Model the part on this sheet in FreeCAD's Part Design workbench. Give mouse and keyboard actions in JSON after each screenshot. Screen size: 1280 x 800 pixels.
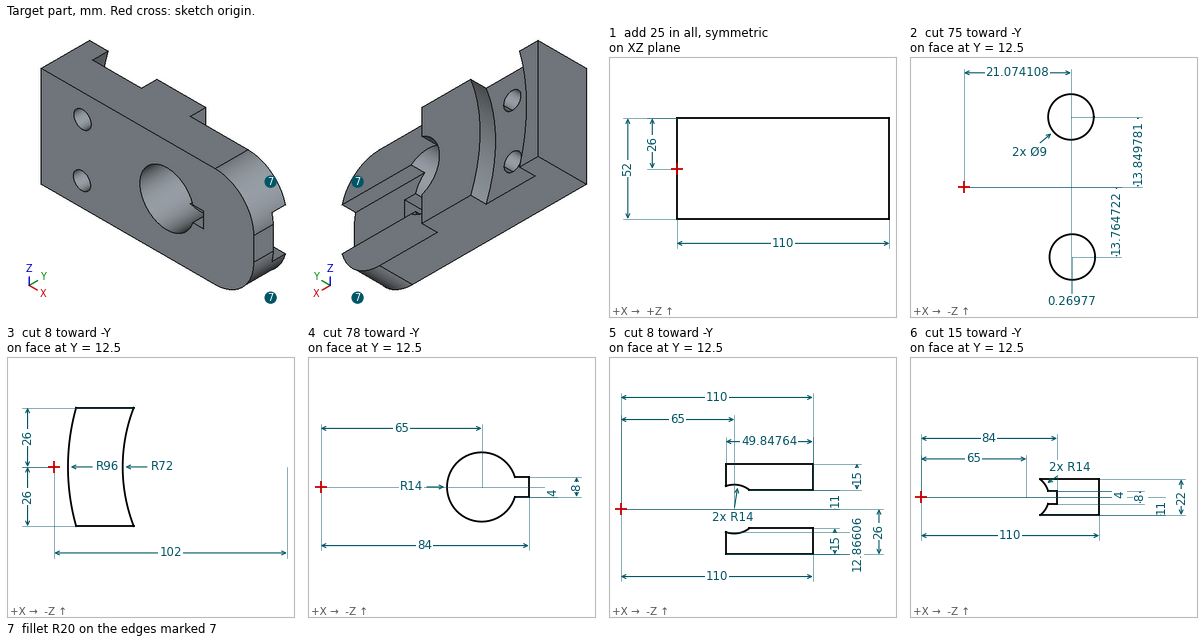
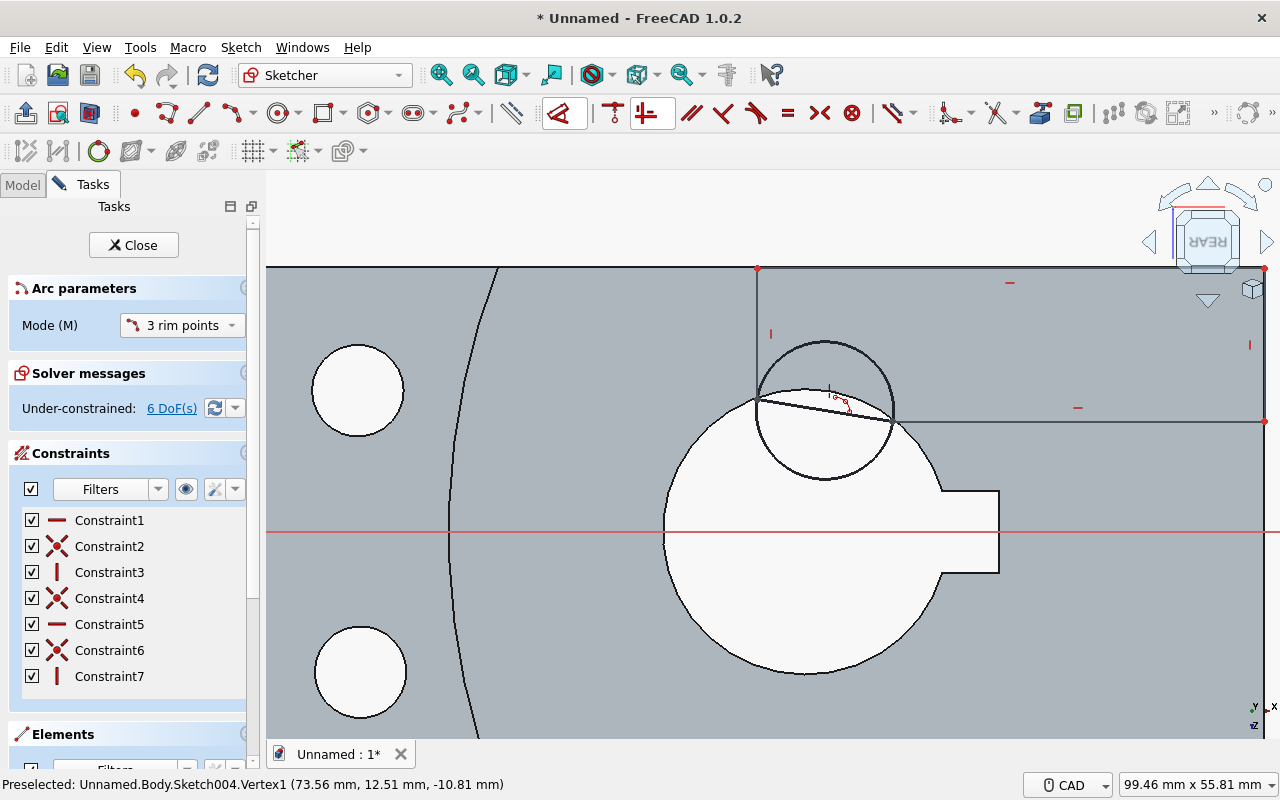
{"action": "left_click", "coordinate": [828, 391]}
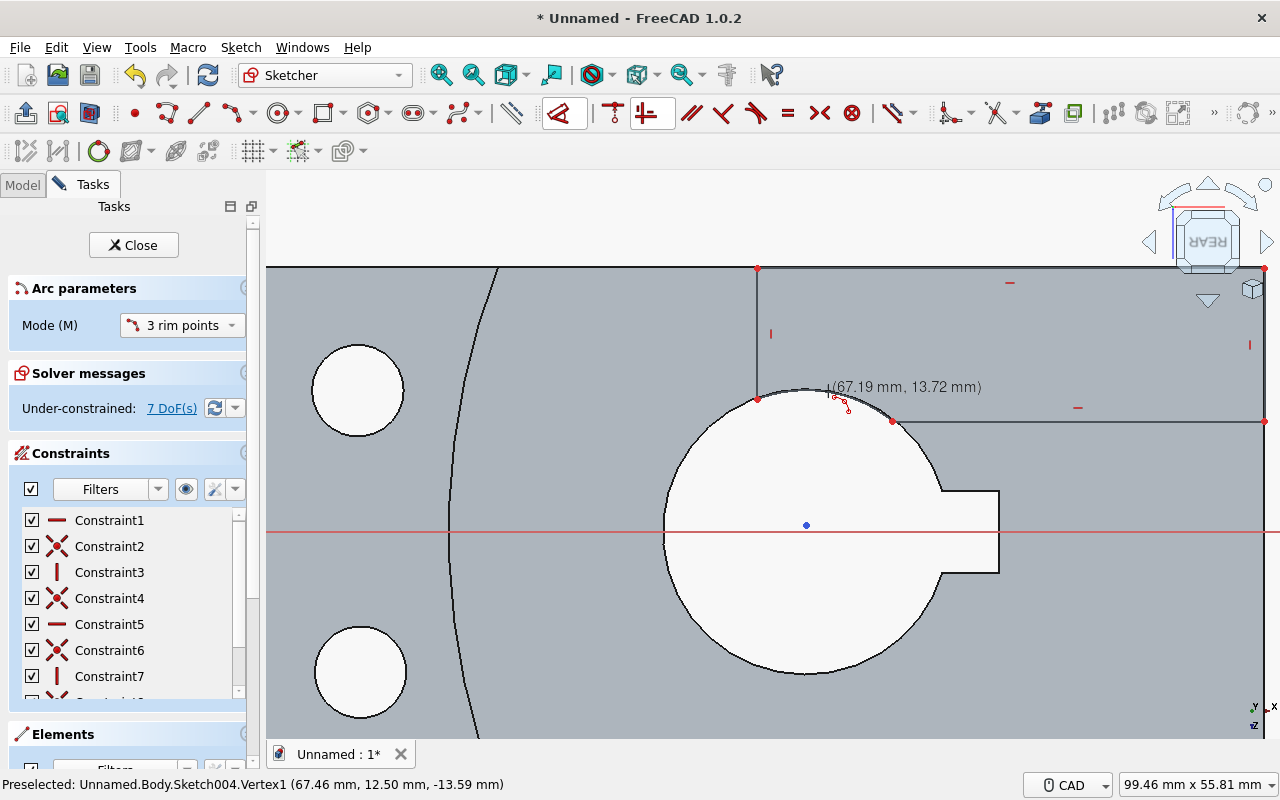
{"action": "left_click", "coordinate": [168, 114]}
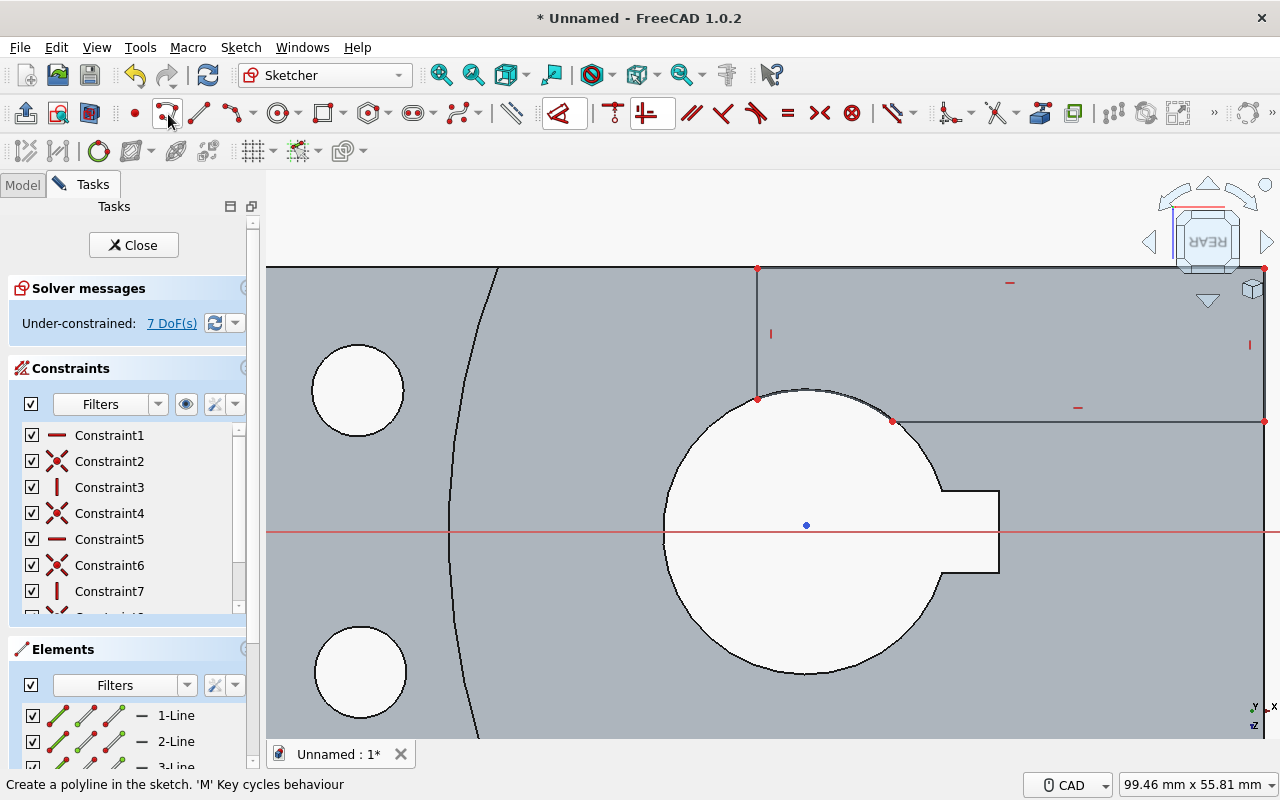
{"action": "left_click", "coordinate": [756, 666]}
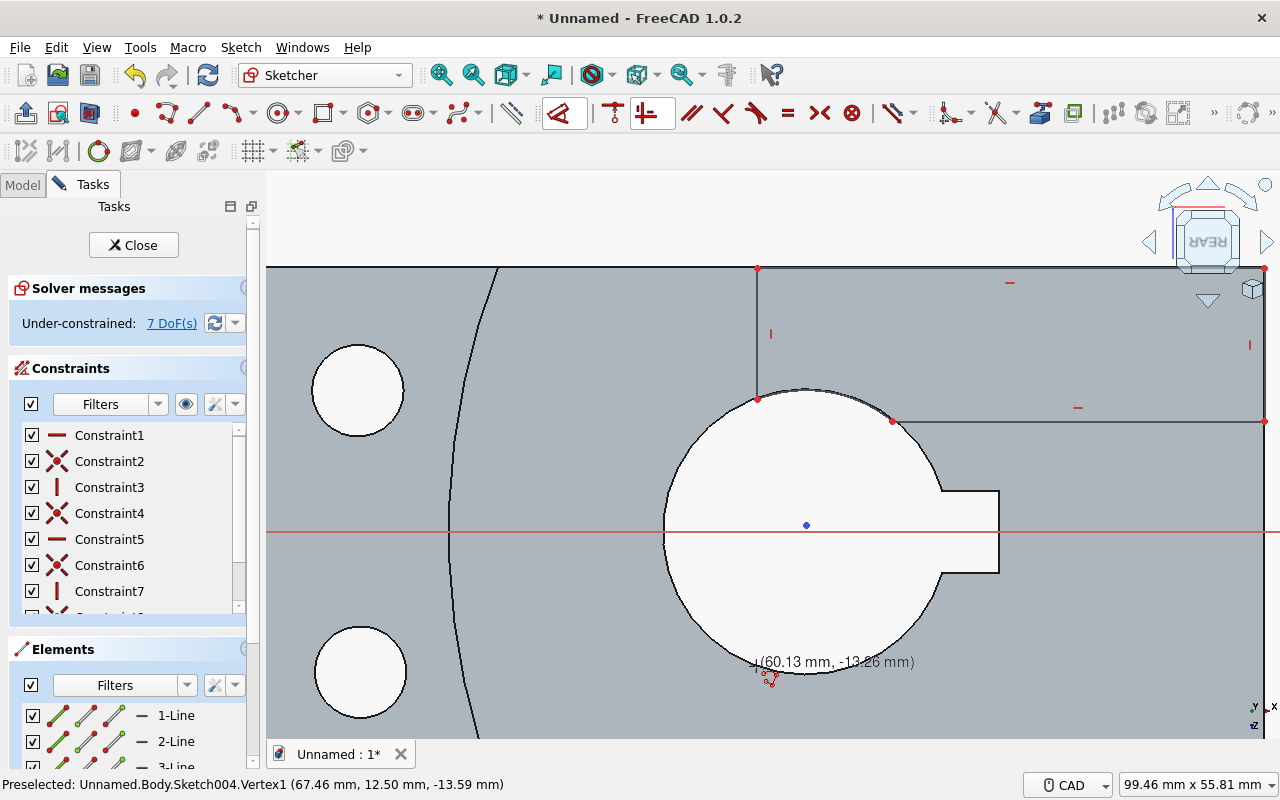
{"action": "scroll", "coordinate": [705, 360], "scroll_direction": "down", "scroll_amount": 3}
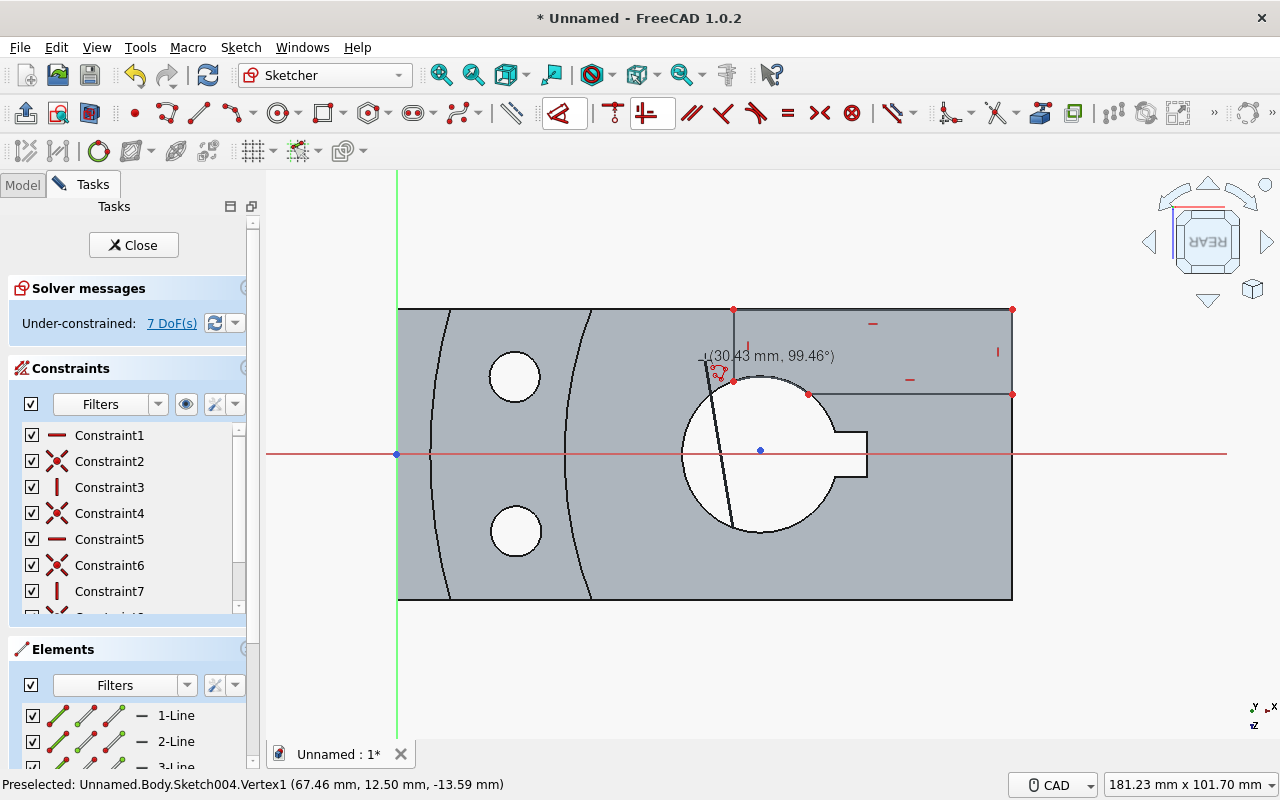
{"action": "left_click", "coordinate": [733, 600]}
{"action": "left_click", "coordinate": [1012, 600]}
{"action": "left_click", "coordinate": [1012, 516]}
{"action": "left_click", "coordinate": [809, 516]}
{"action": "right_click", "coordinate": [809, 516]}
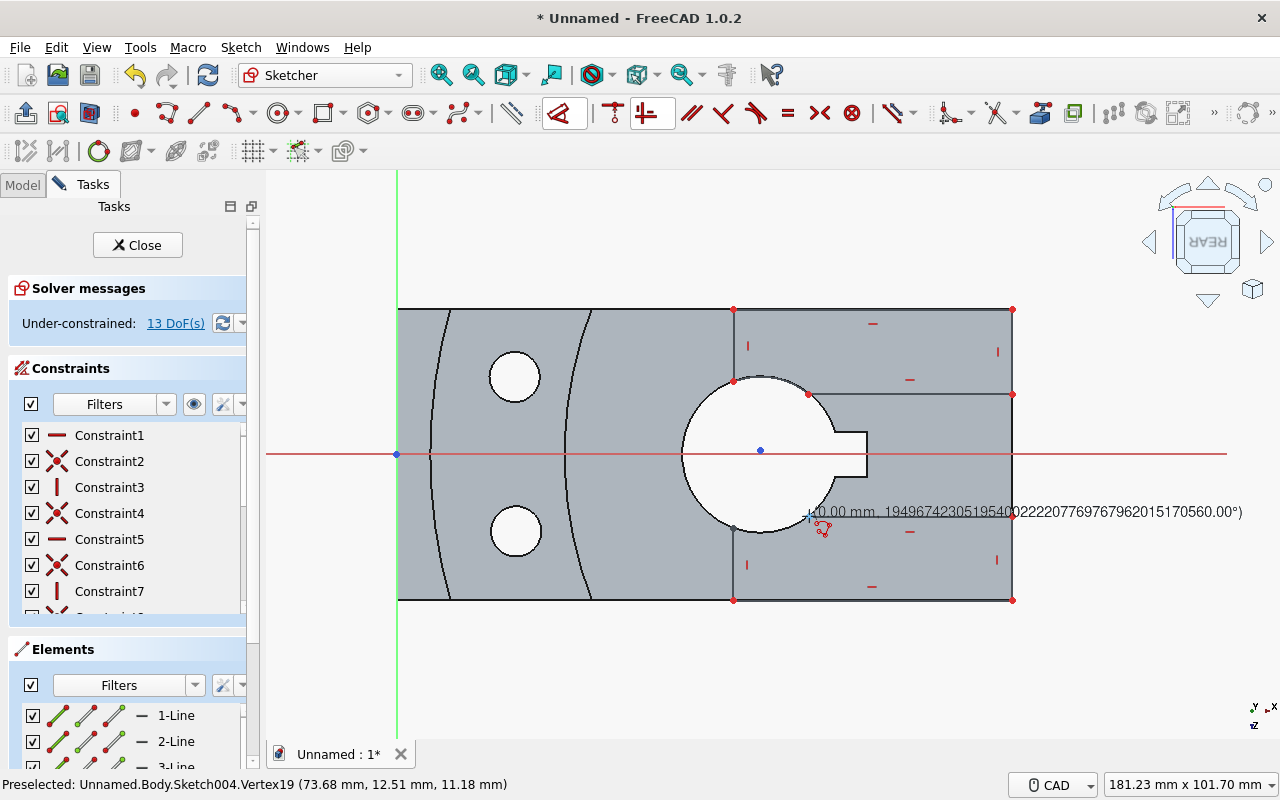
{"action": "left_click", "coordinate": [232, 114]}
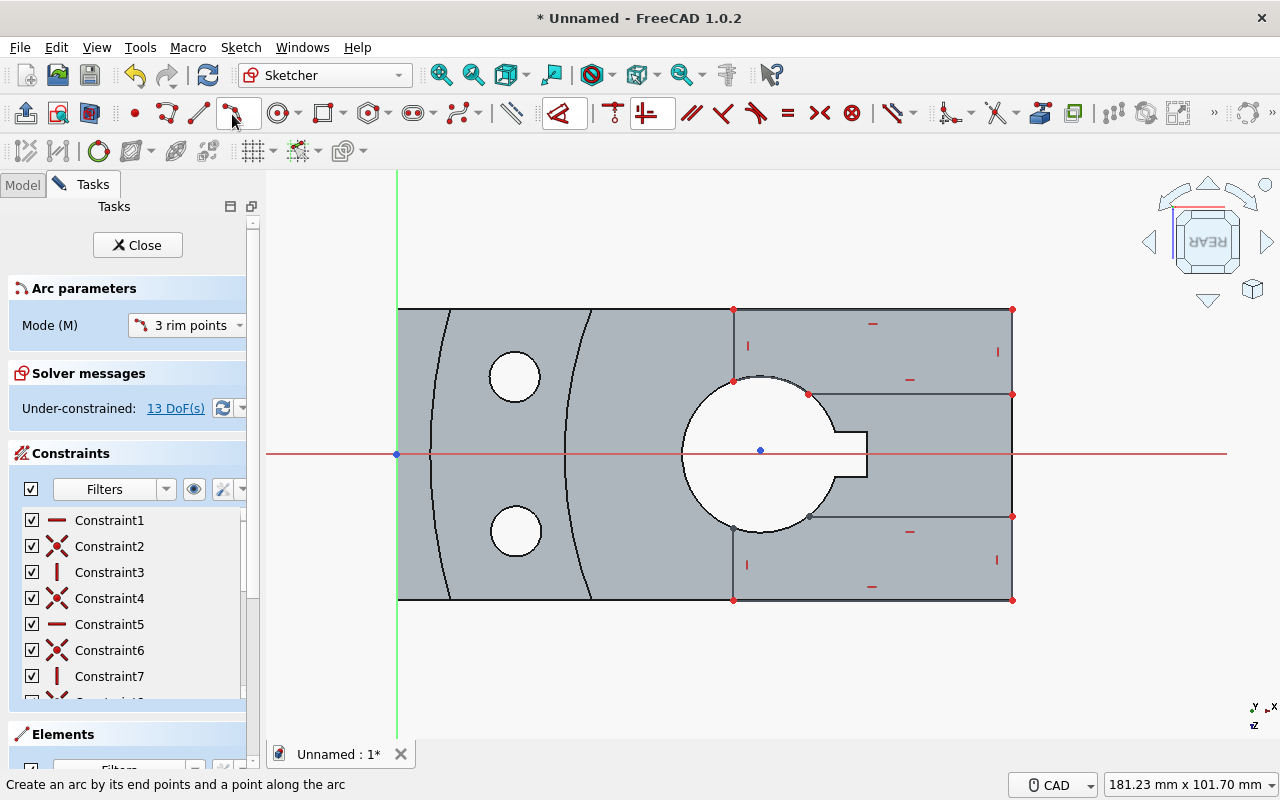
{"action": "left_click", "coordinate": [809, 517]}
{"action": "left_click", "coordinate": [733, 529]}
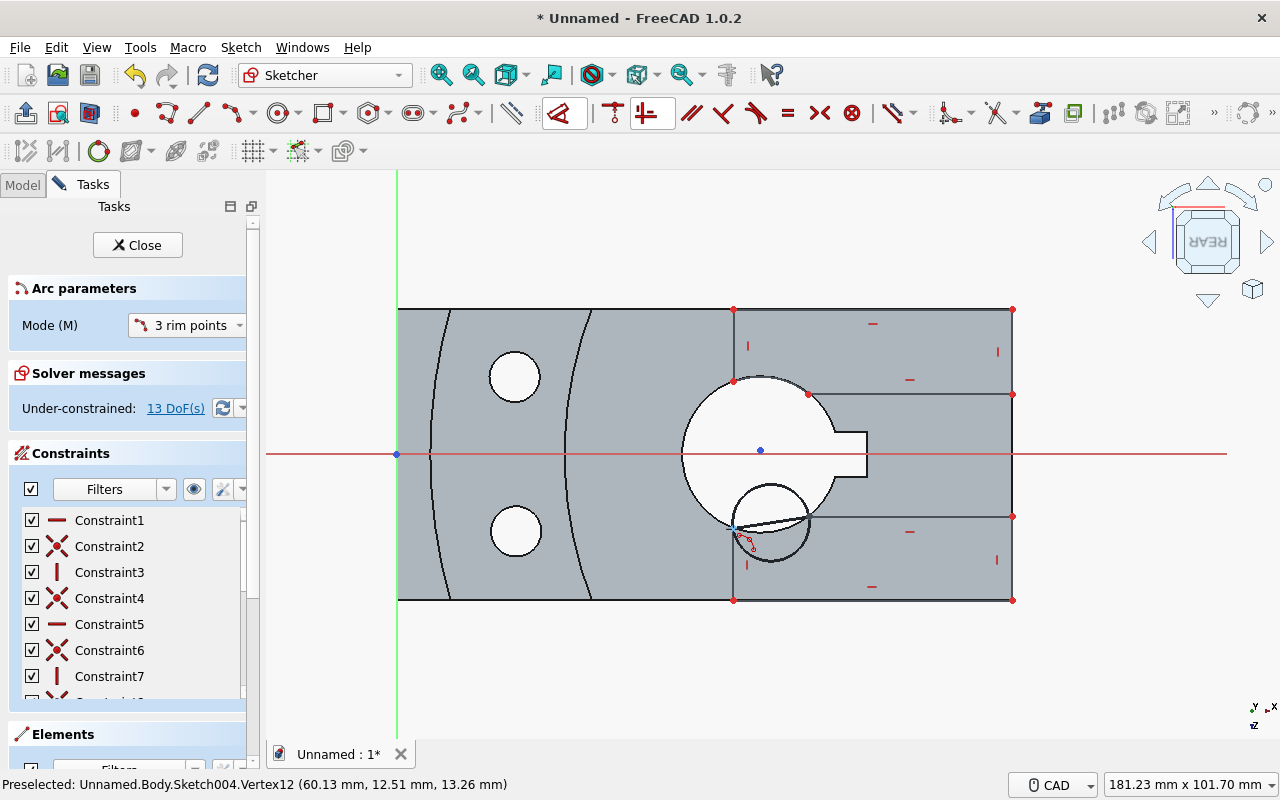
{"action": "scroll", "coordinate": [773, 532], "scroll_direction": "up", "scroll_amount": 3}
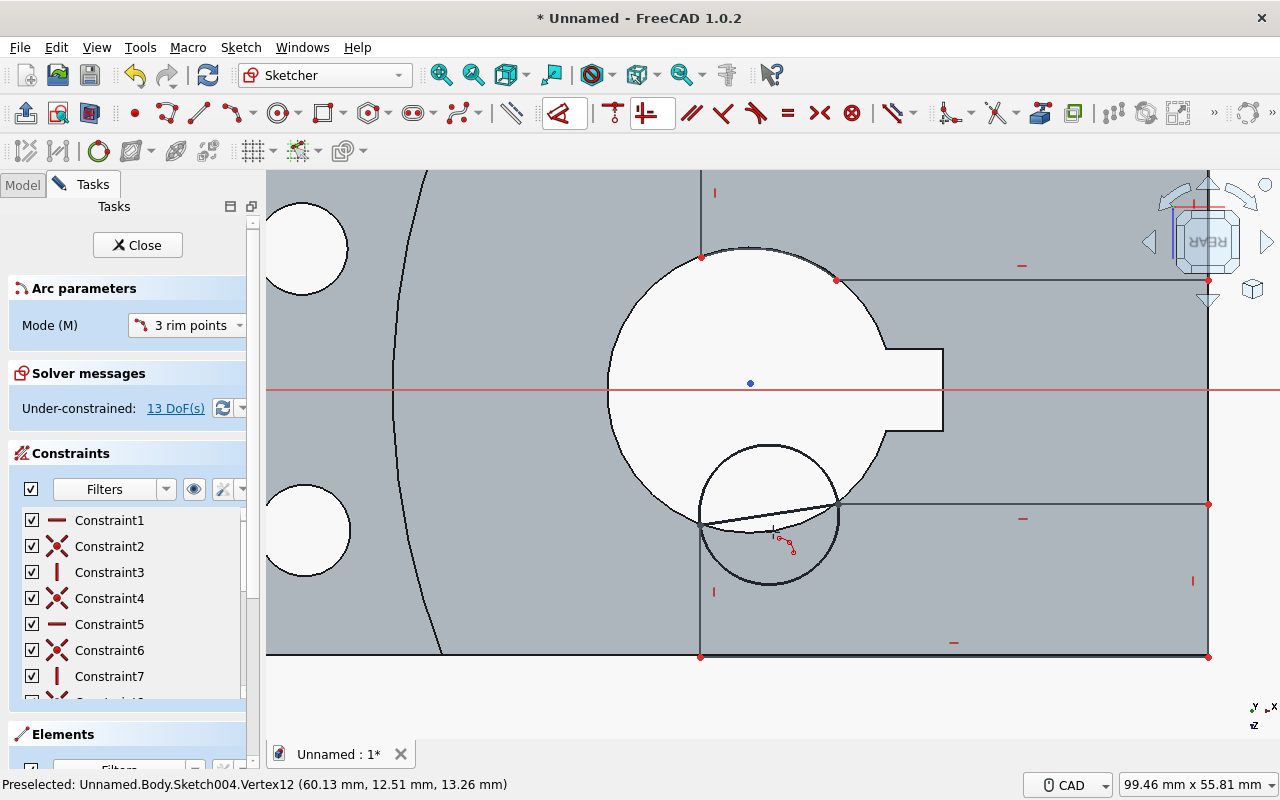
{"action": "left_click", "coordinate": [772, 531]}
{"action": "key", "text": "Escape"}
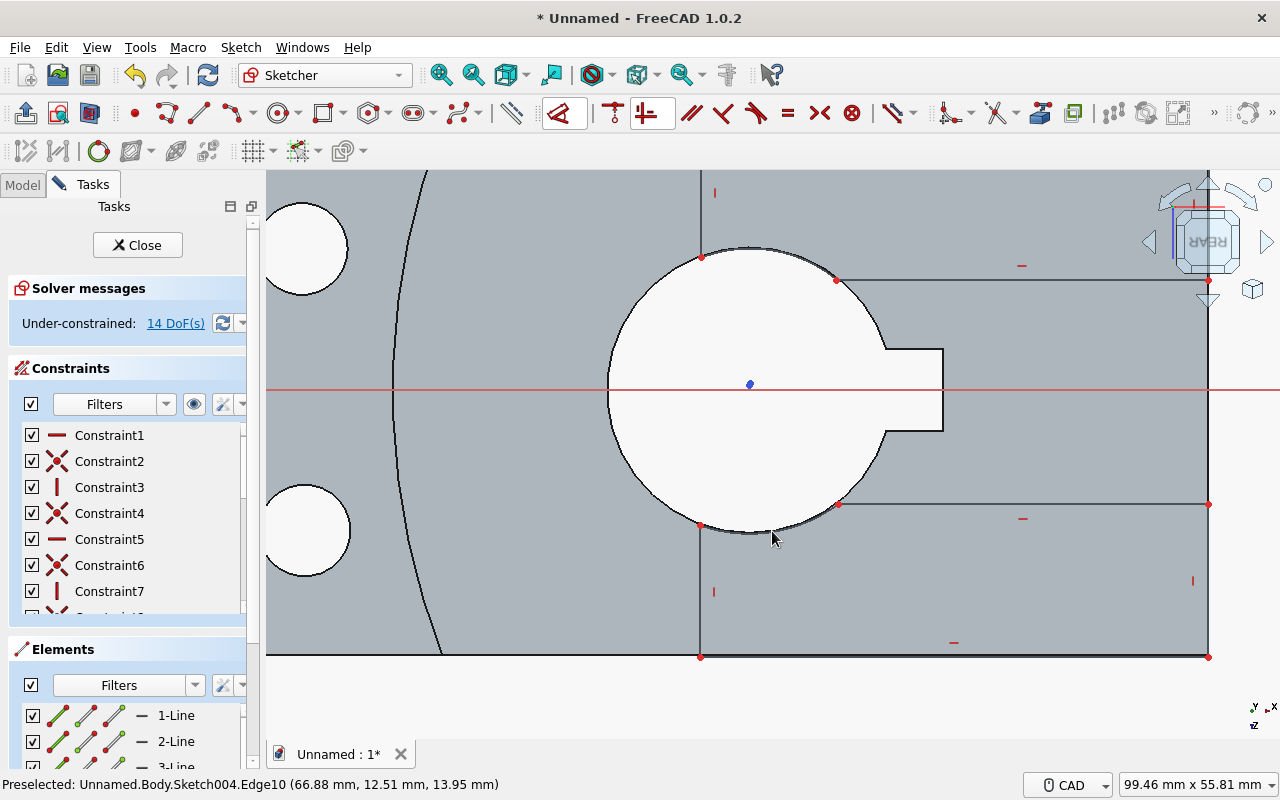
{"action": "left_click", "coordinate": [800, 258]}